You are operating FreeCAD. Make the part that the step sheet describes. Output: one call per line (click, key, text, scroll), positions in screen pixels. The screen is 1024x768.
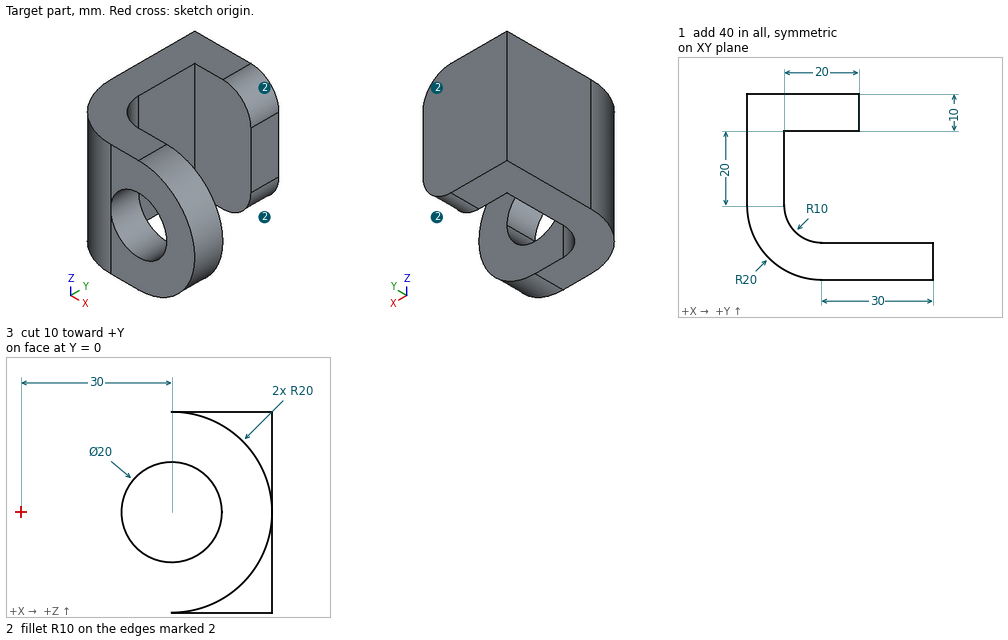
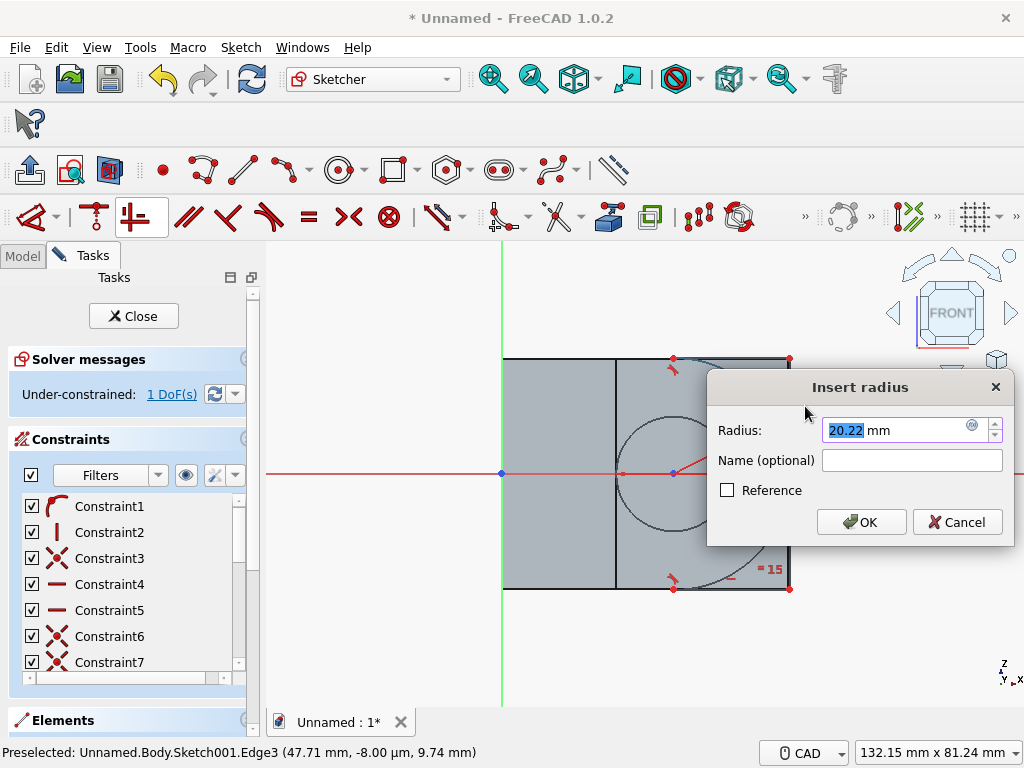
text(20)
key(Return)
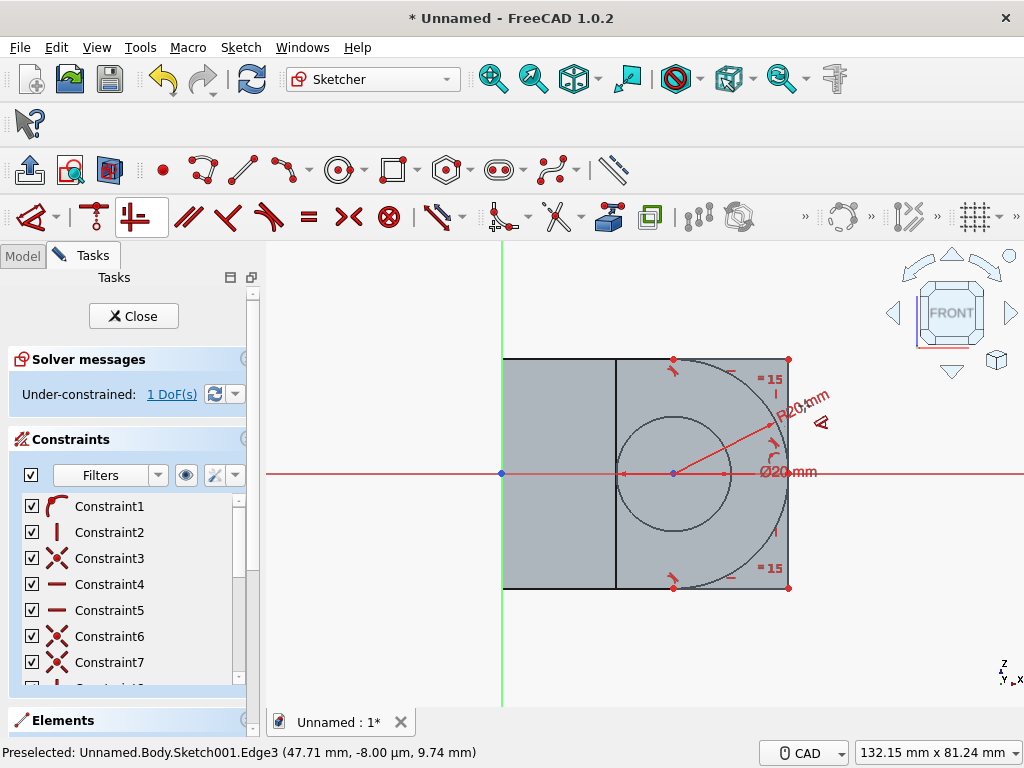
click(674, 474)
click(588, 508)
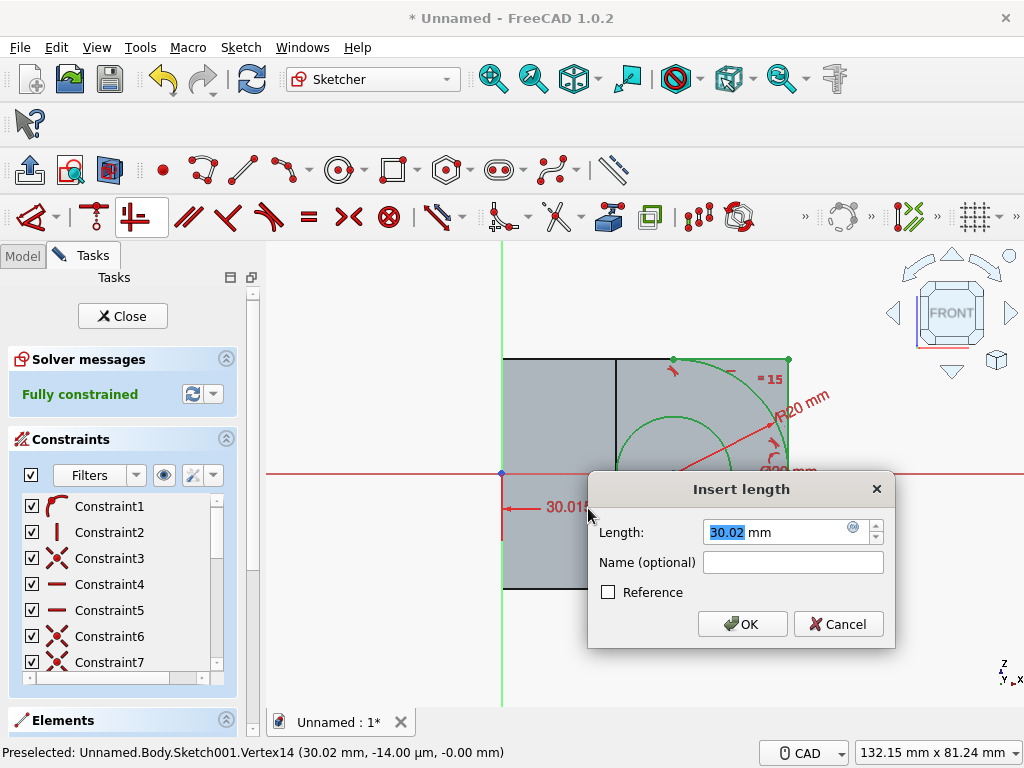
text(30)
key(Return)
key(Escape)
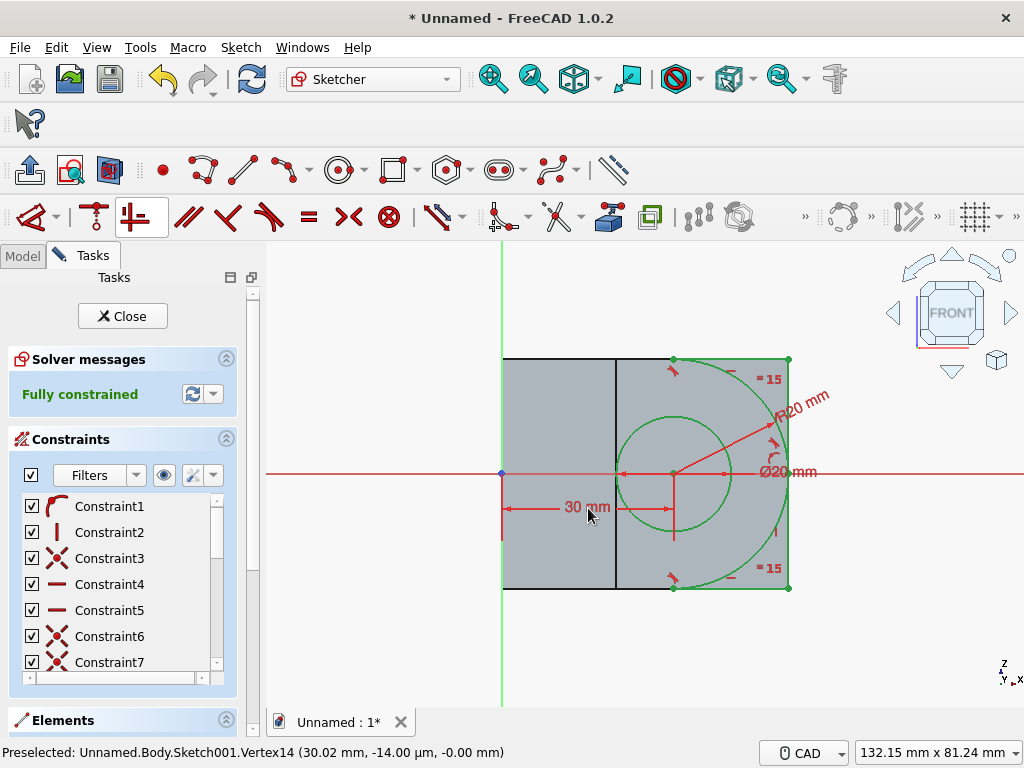
click(123, 316)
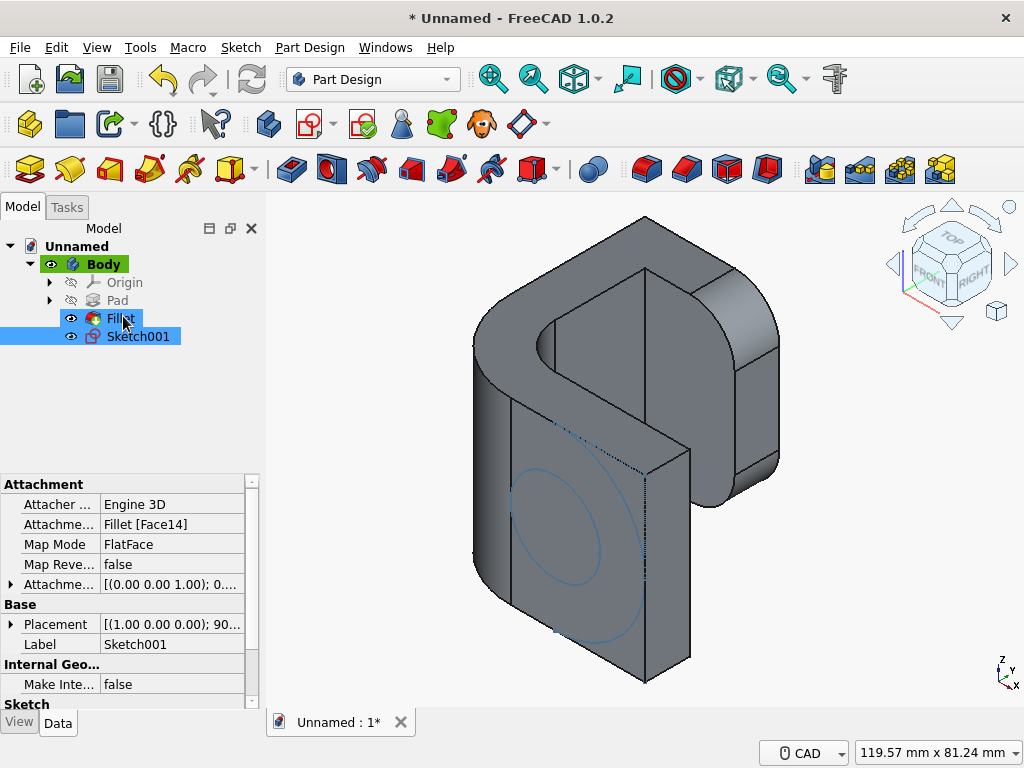
click(292, 170)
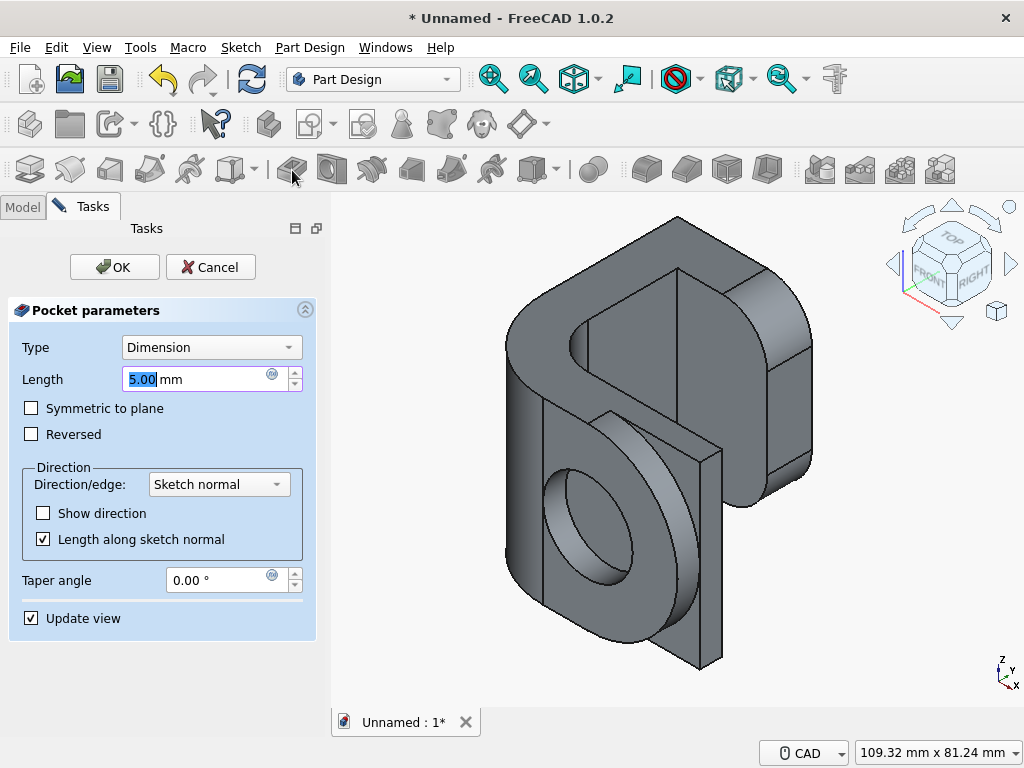
text(10)
key(Tab)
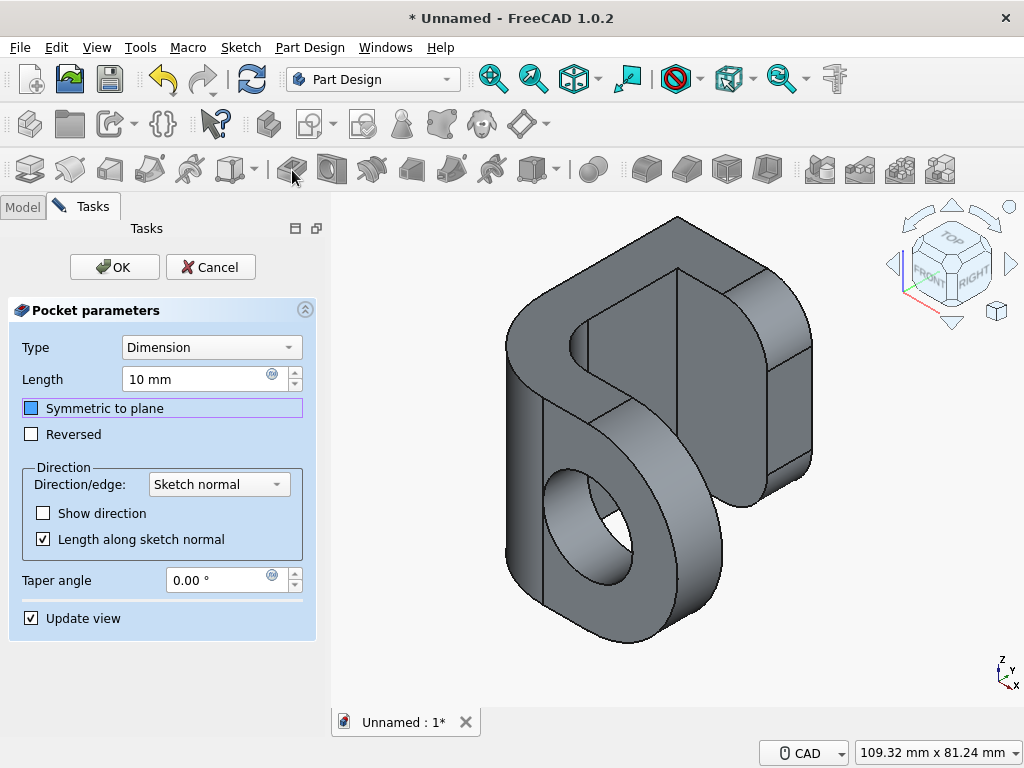
click(115, 267)